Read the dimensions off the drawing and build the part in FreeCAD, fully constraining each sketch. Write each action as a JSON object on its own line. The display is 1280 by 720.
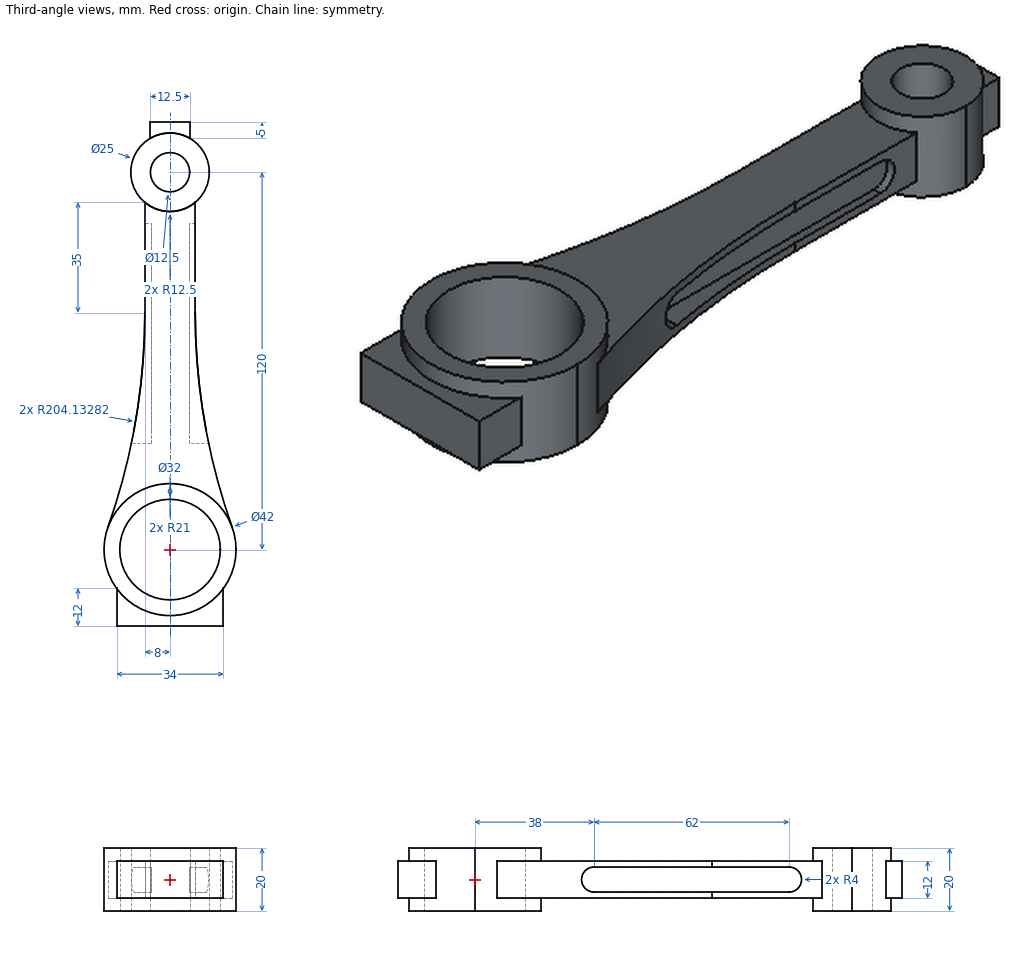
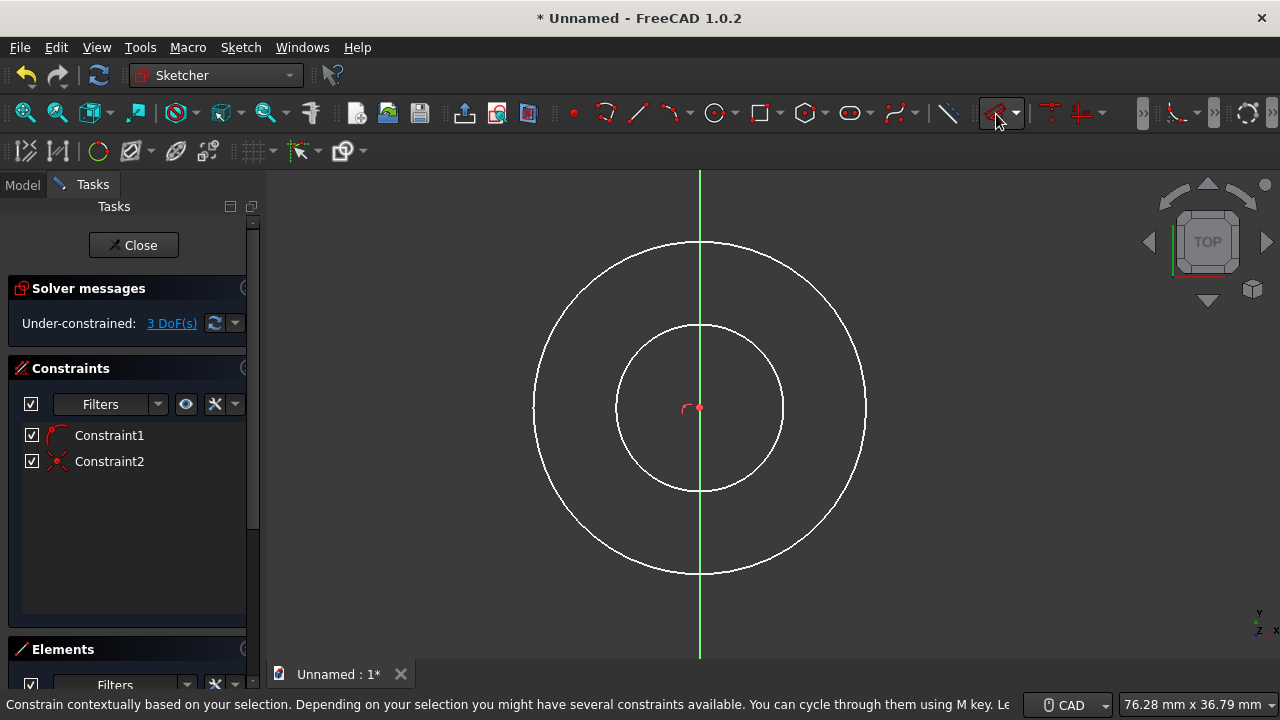
{"action": "left_click", "coordinate": [817, 290]}
{"action": "left_click", "coordinate": [840, 267]}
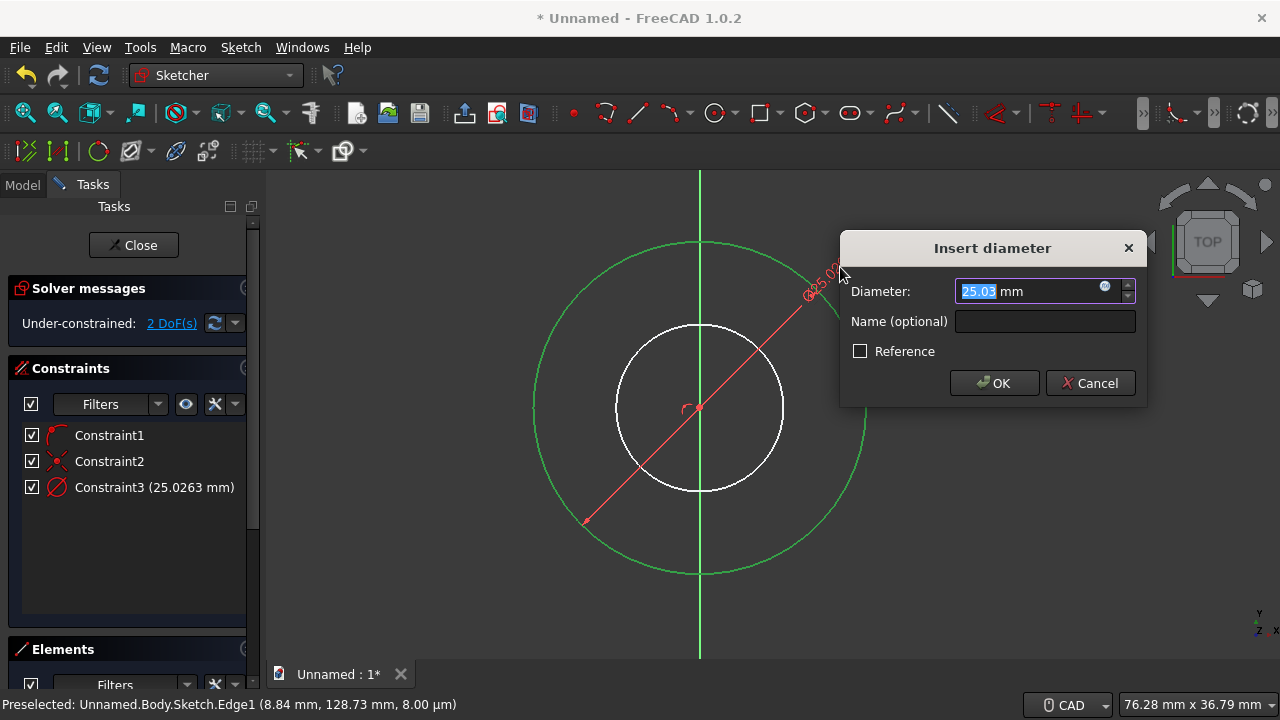
{"action": "type", "text": "25"}
{"action": "key", "text": "Return"}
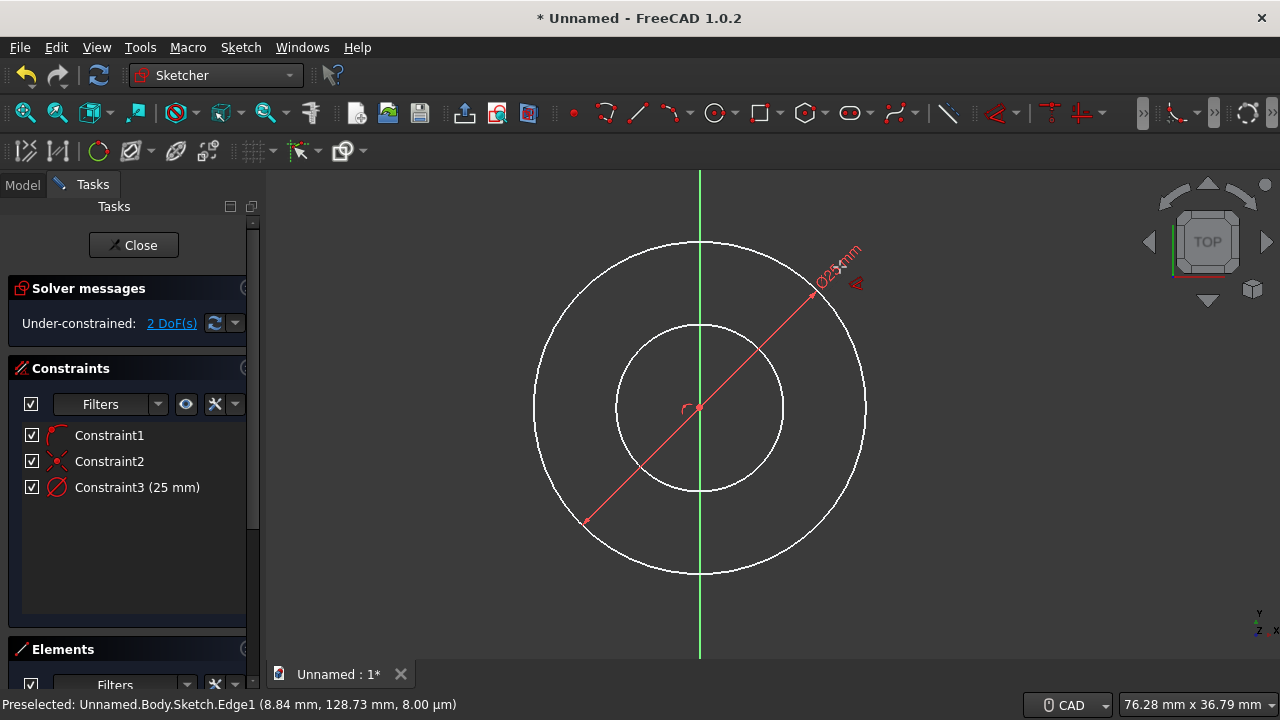
{"action": "left_click", "coordinate": [759, 349]}
{"action": "left_click", "coordinate": [782, 326]}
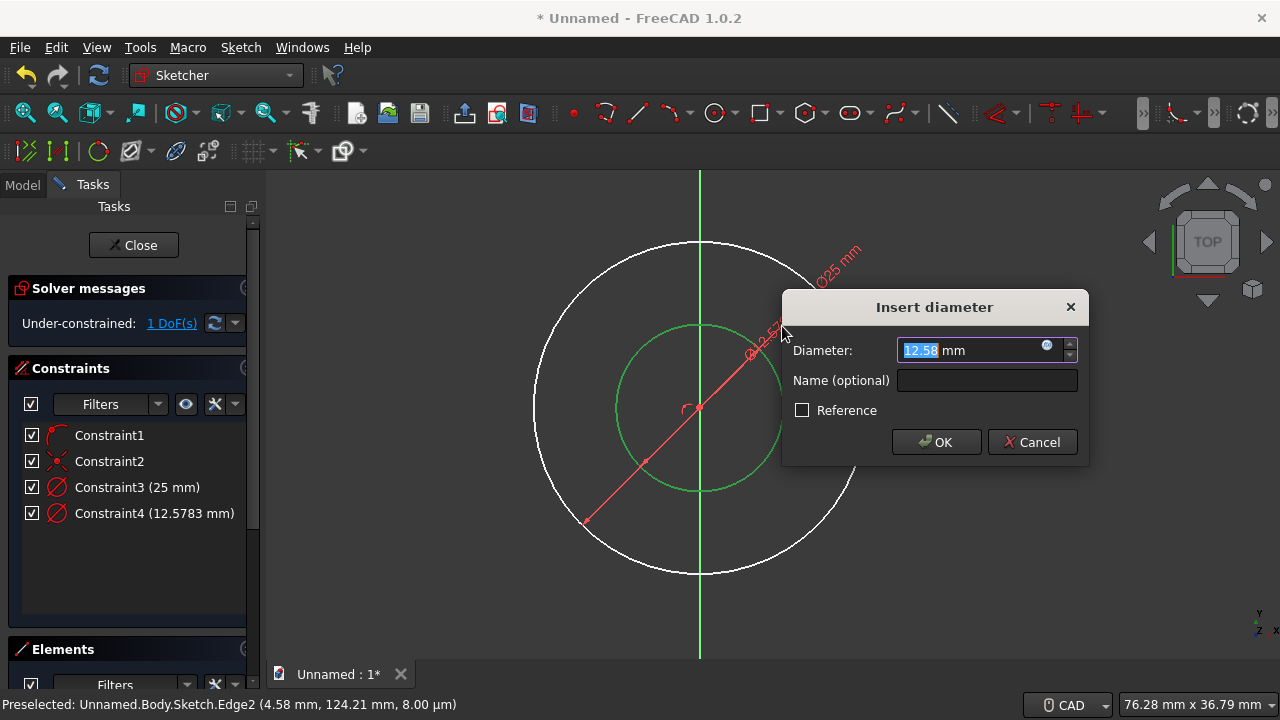
{"action": "type", "text": "12.5"}
{"action": "key", "text": "Return"}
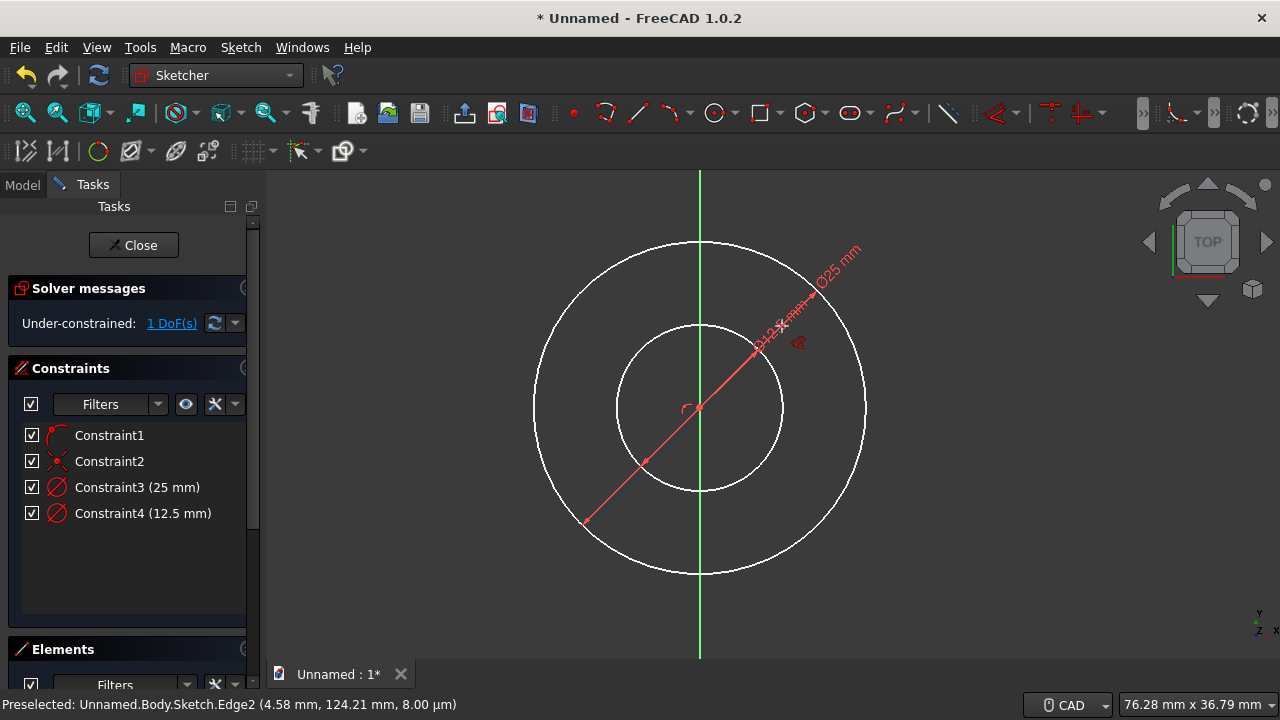
{"action": "left_click", "coordinate": [700, 408]}
{"action": "left_click", "coordinate": [734, 520]}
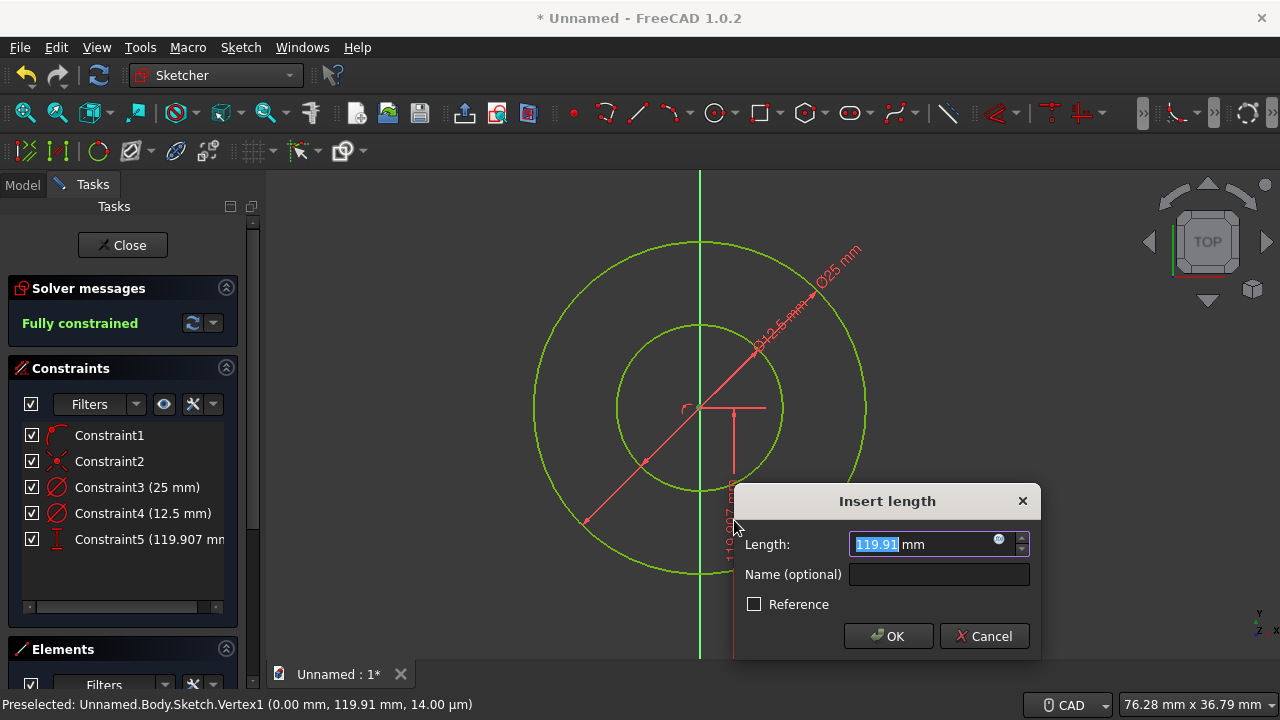
{"action": "type", "text": "120"}
{"action": "key", "text": "Return"}
{"action": "key", "text": "Escape"}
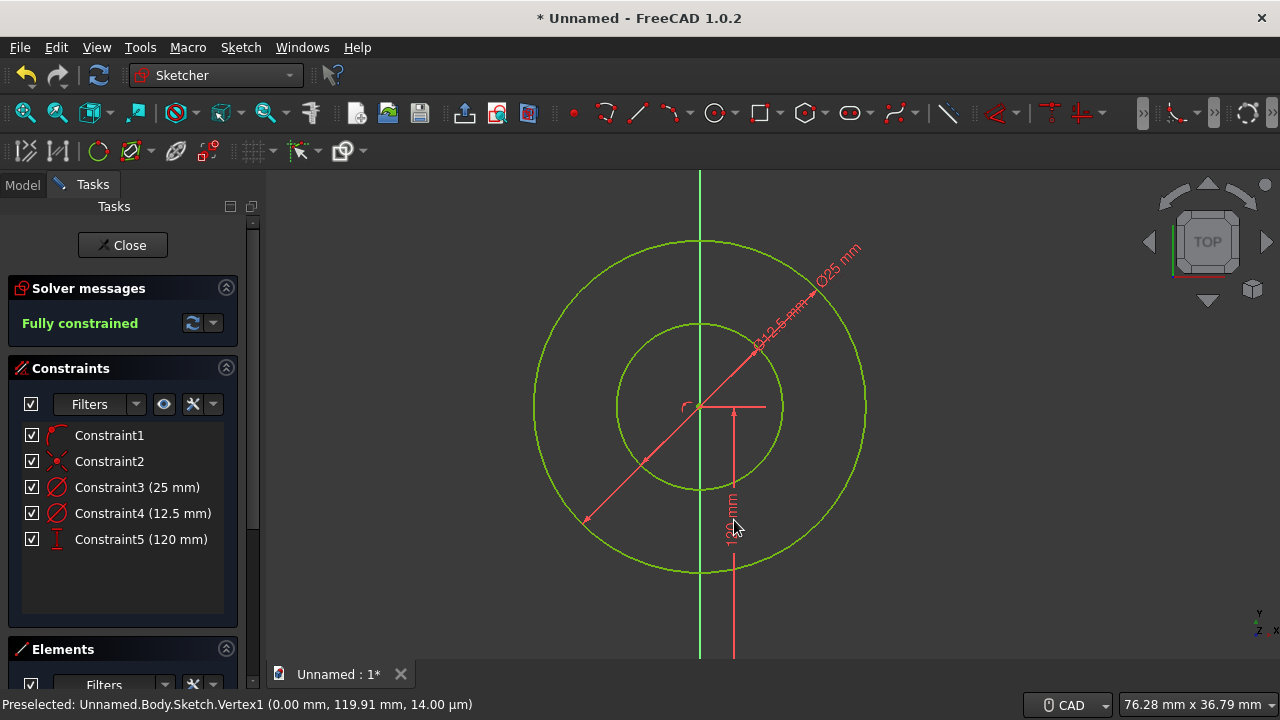
{"action": "left_click", "coordinate": [123, 245]}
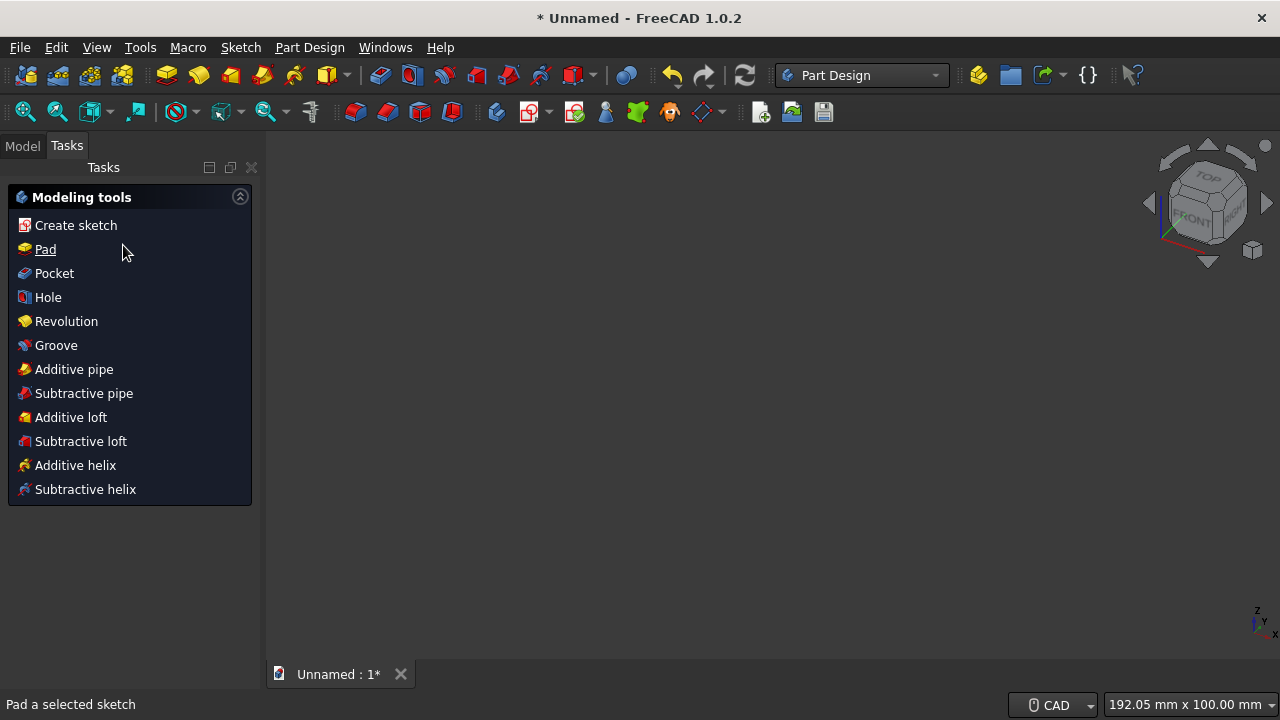
{"action": "left_click", "coordinate": [168, 76]}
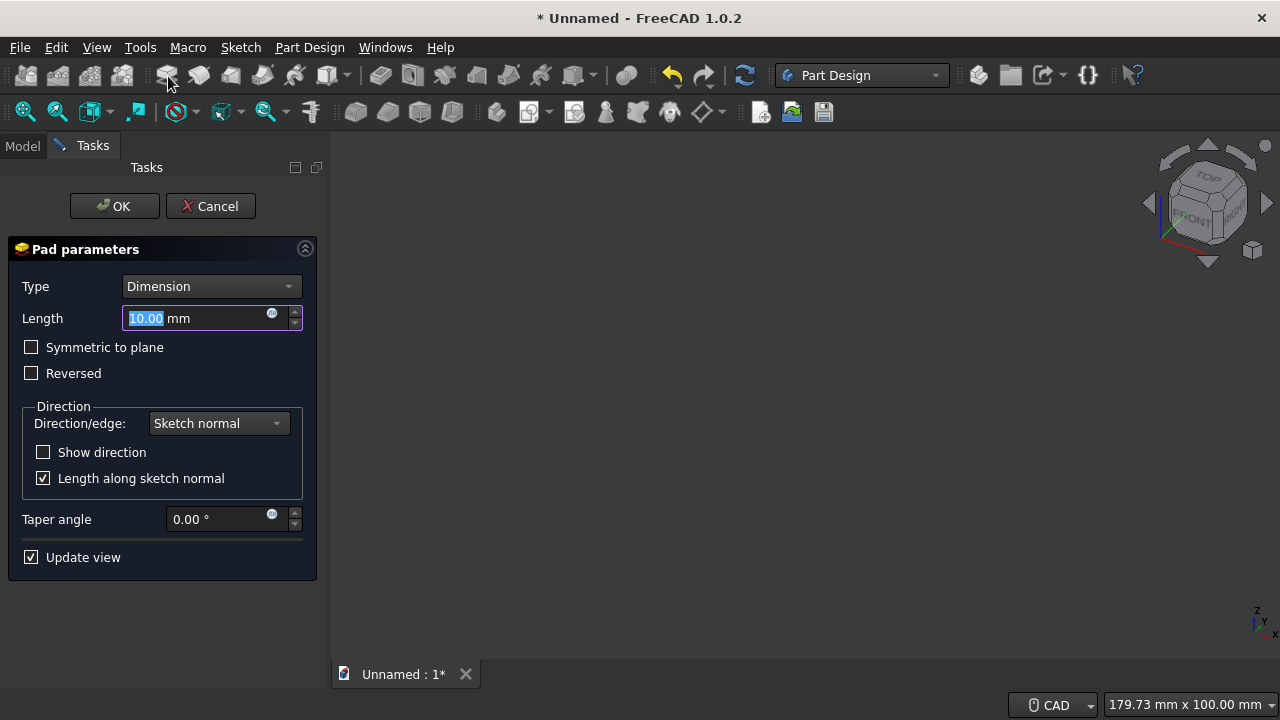
{"action": "type", "text": "20"}
{"action": "key", "text": "Tab"}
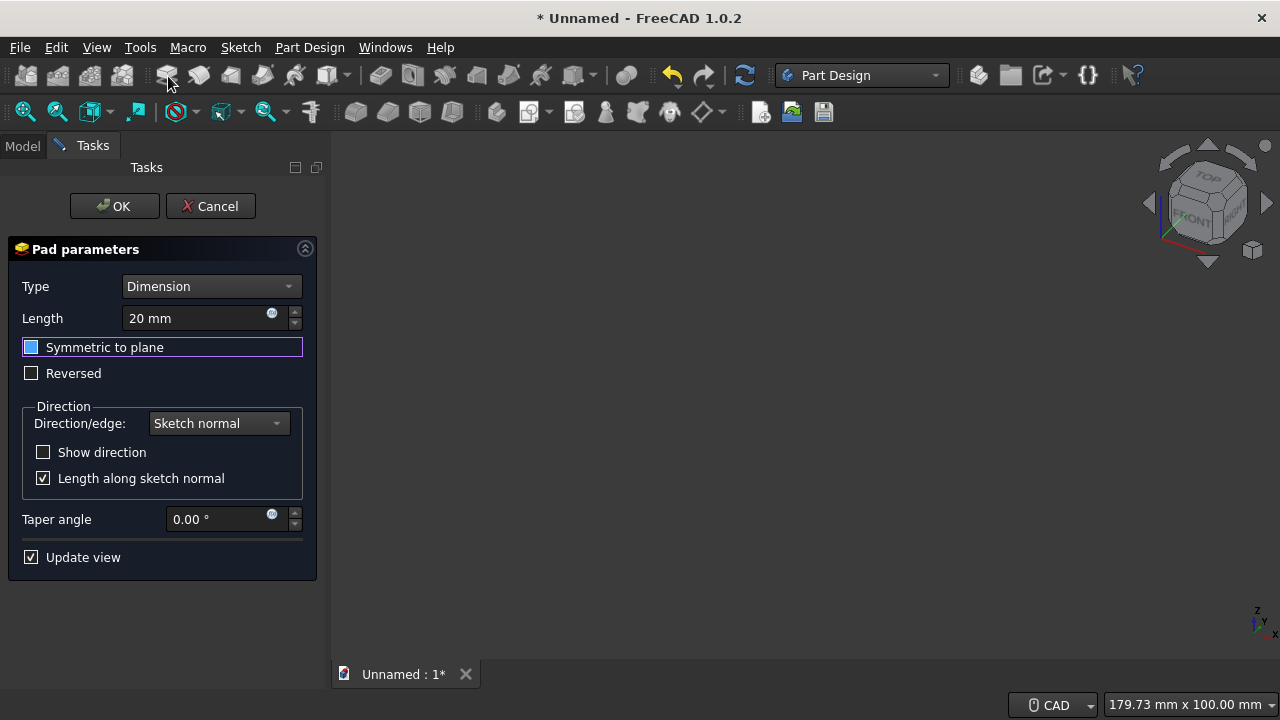
{"action": "left_click", "coordinate": [30, 347]}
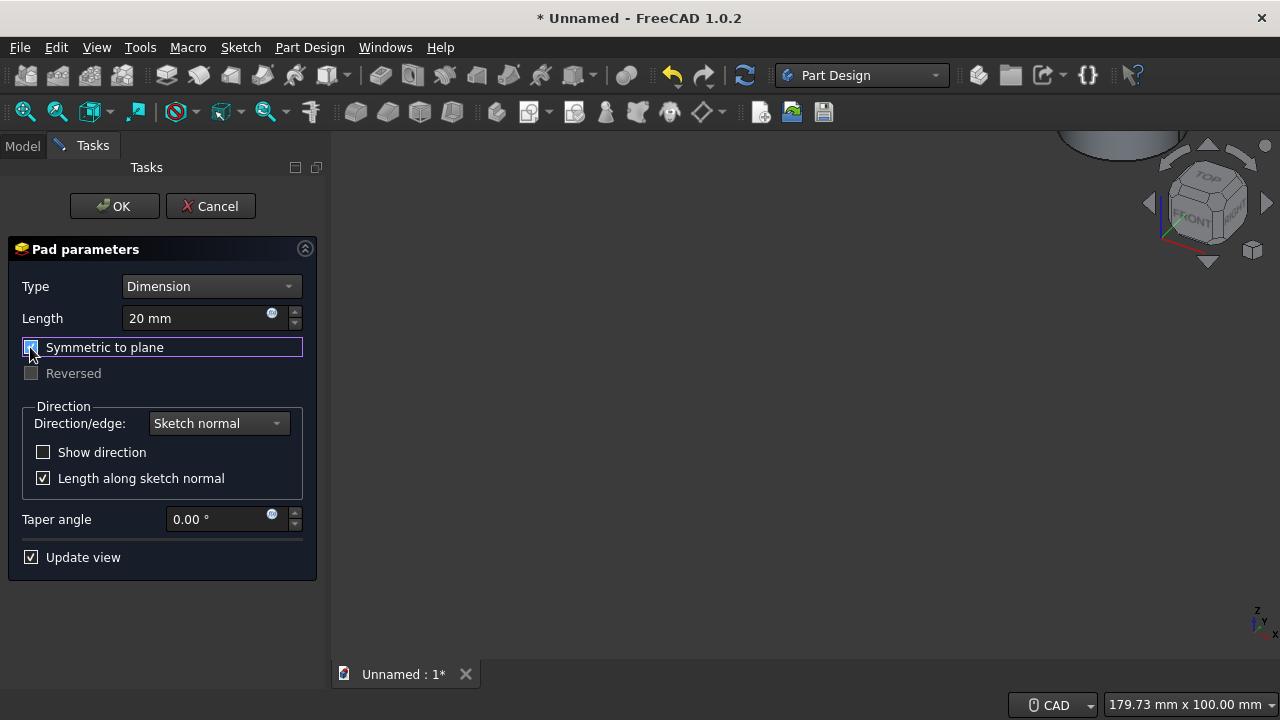
{"action": "left_click", "coordinate": [115, 206]}